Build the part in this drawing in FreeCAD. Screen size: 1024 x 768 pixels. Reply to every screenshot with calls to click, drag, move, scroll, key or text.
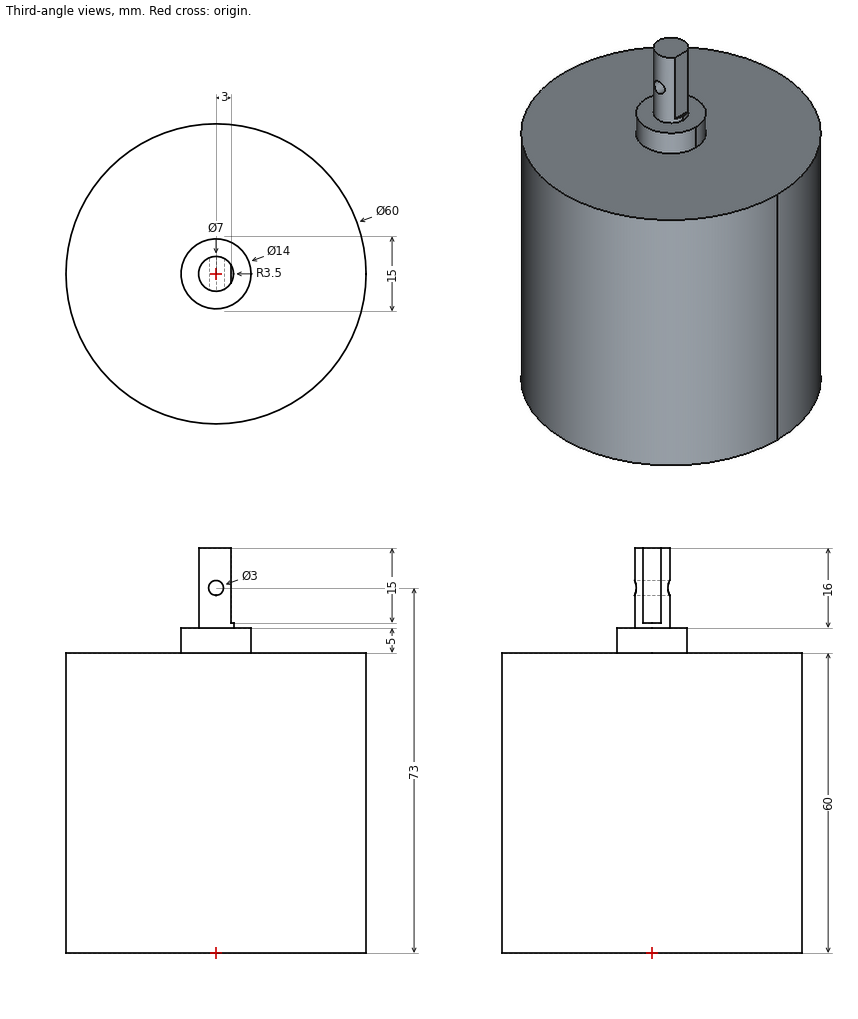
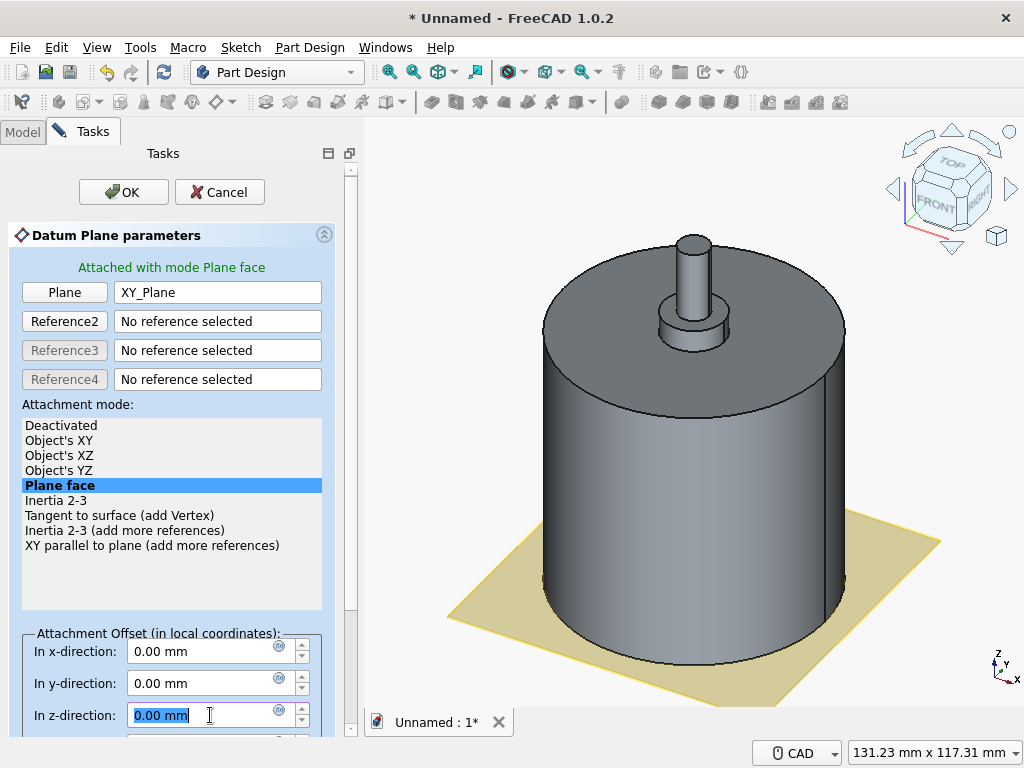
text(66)
key(Tab)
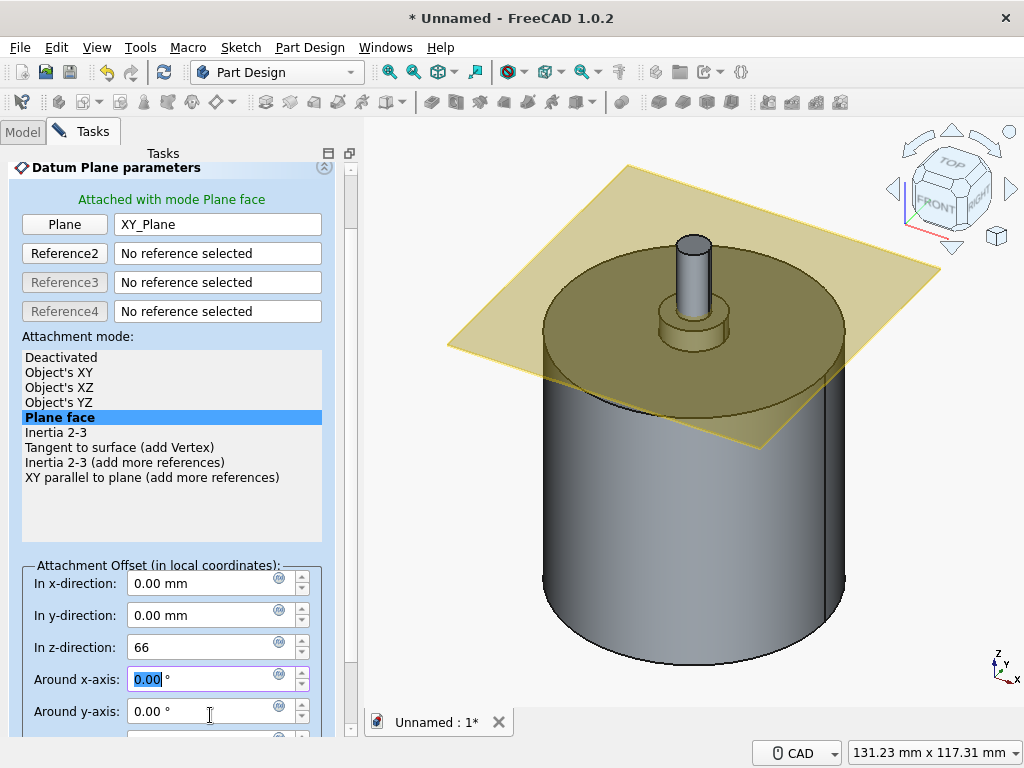
scroll(351, 450, up, 2)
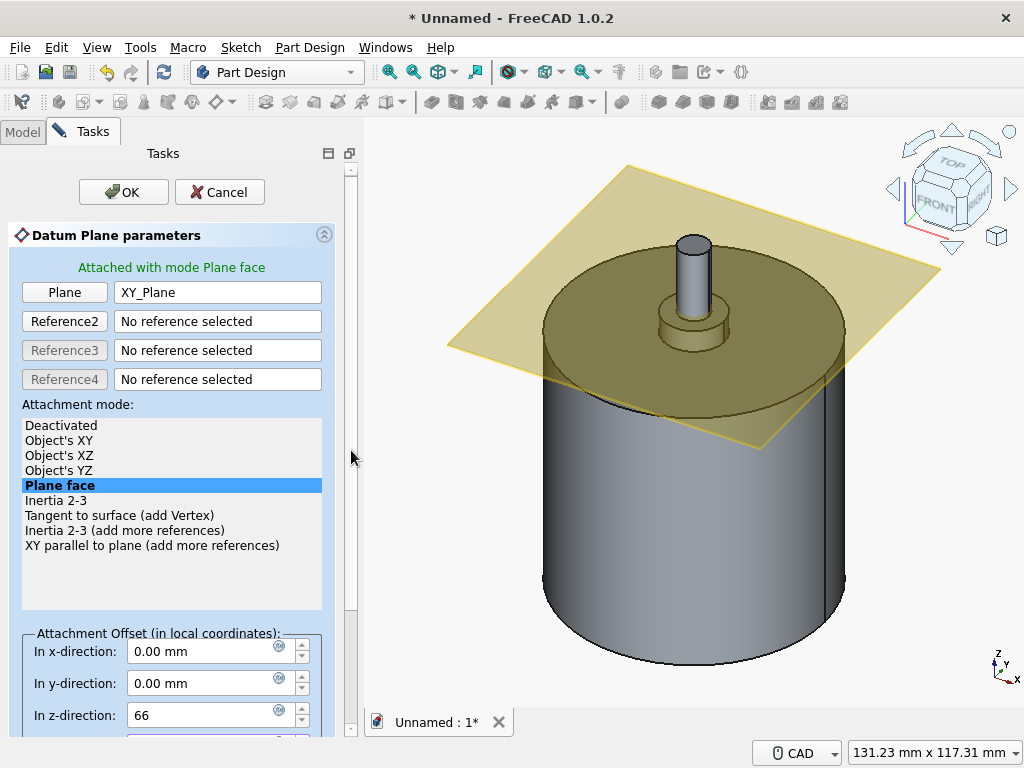
click(124, 192)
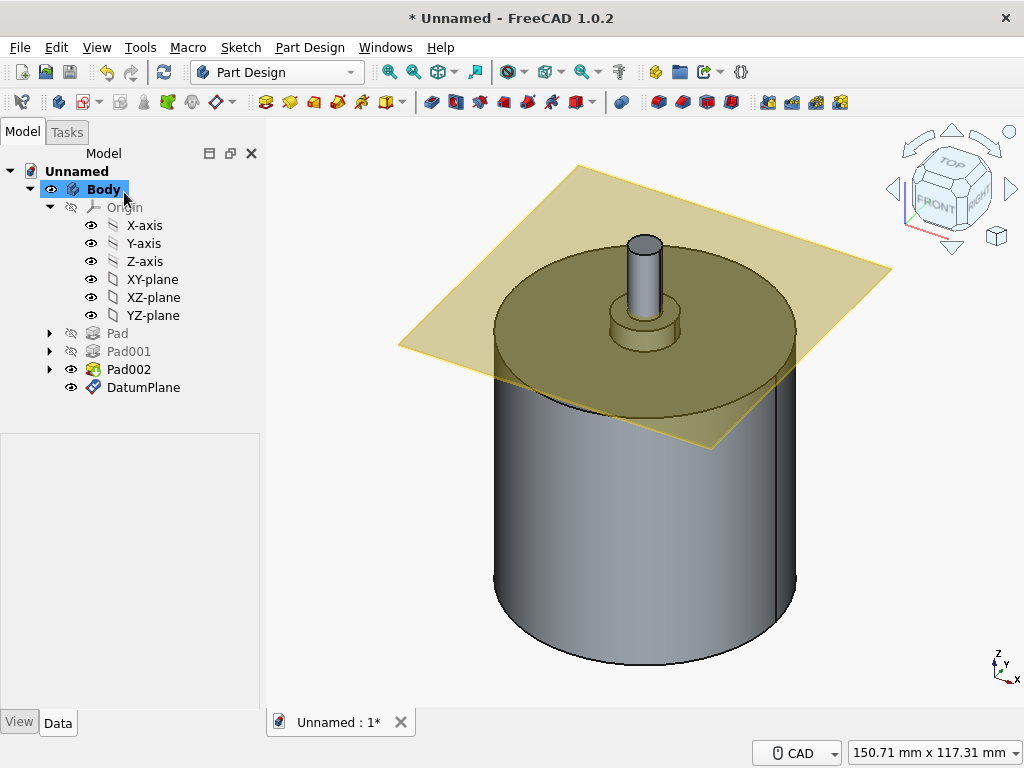
click(116, 387)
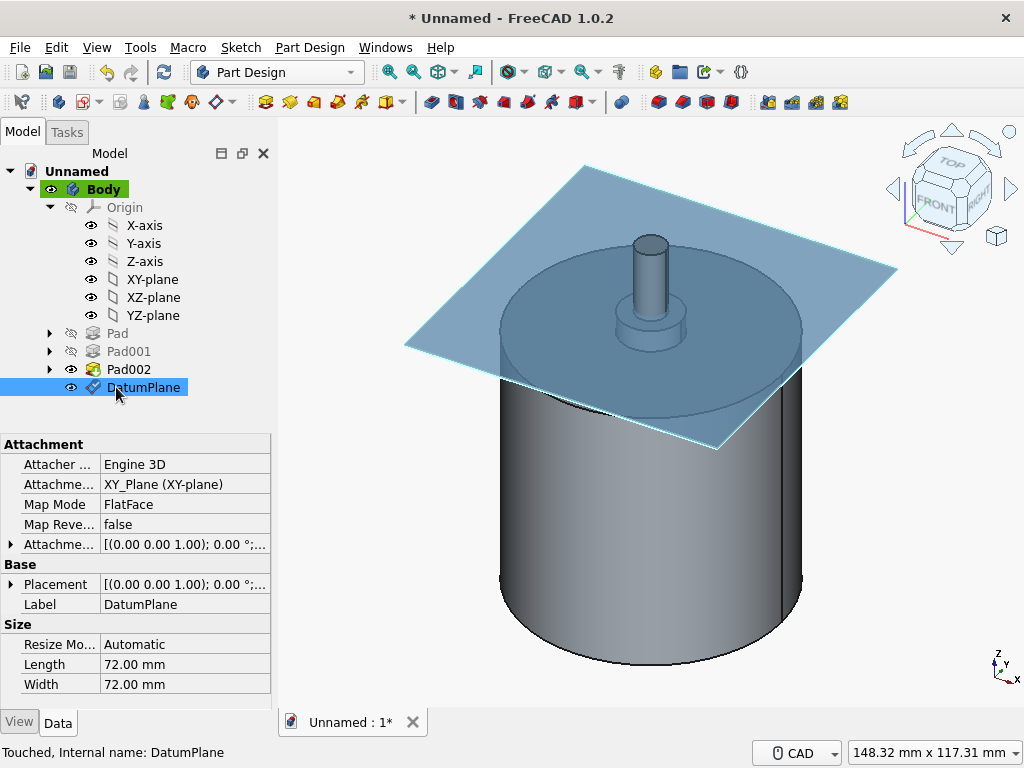
click(84, 102)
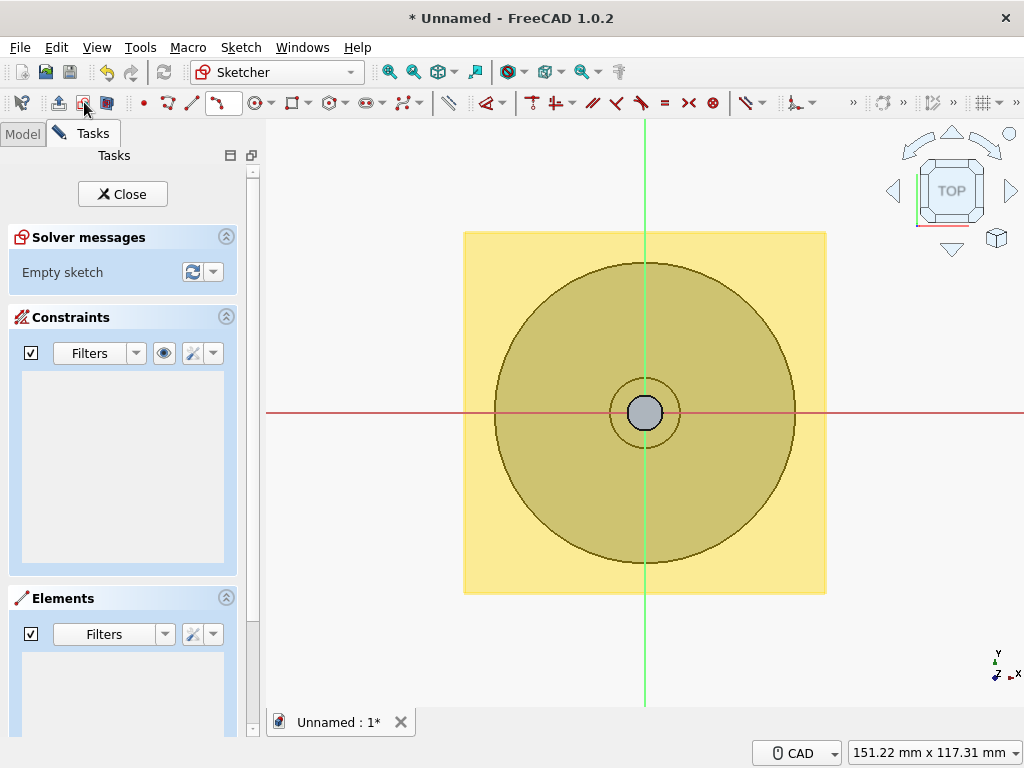
click(108, 104)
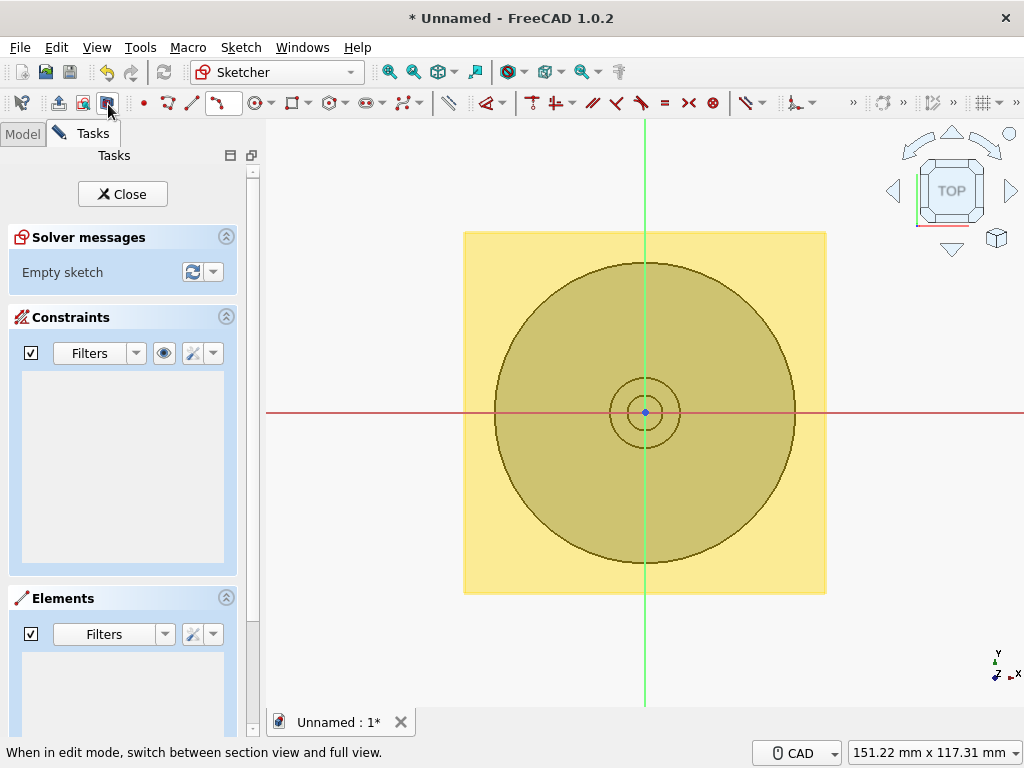
scroll(658, 413, up, 15)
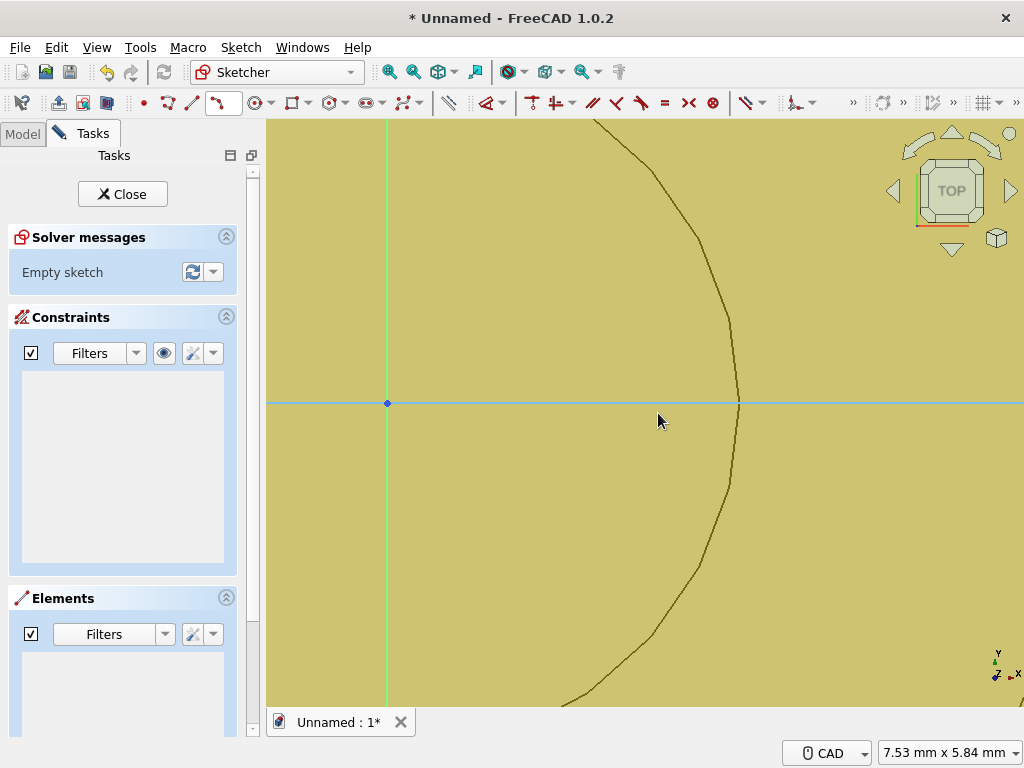
click(192, 104)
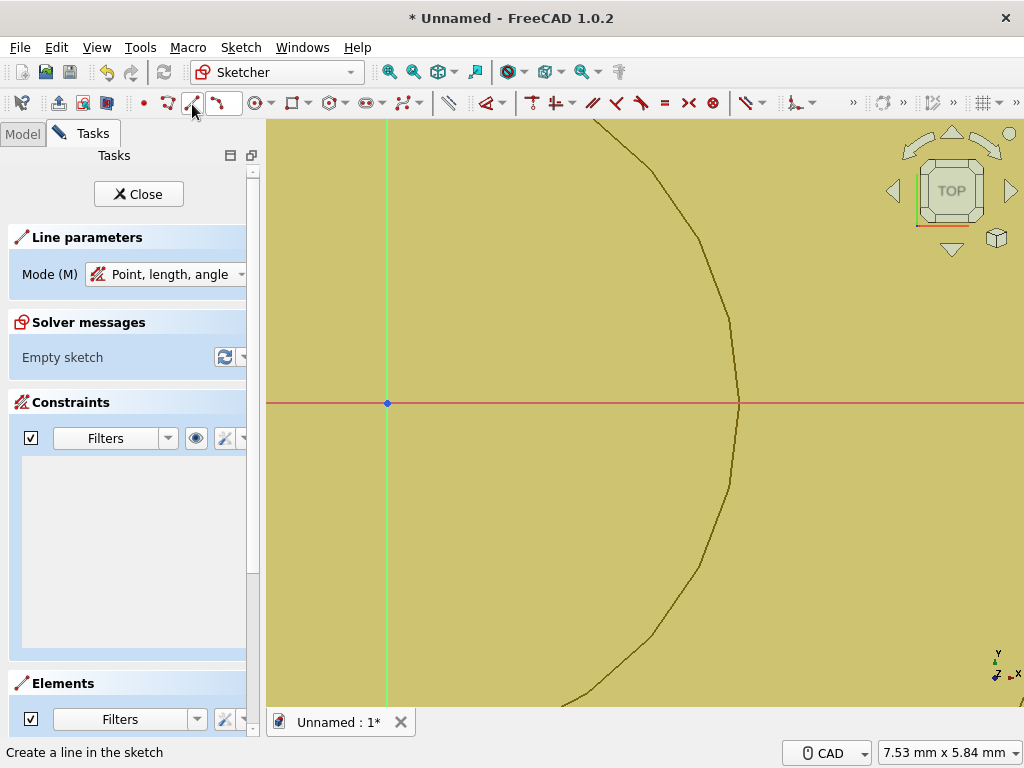
click(689, 222)
click(689, 585)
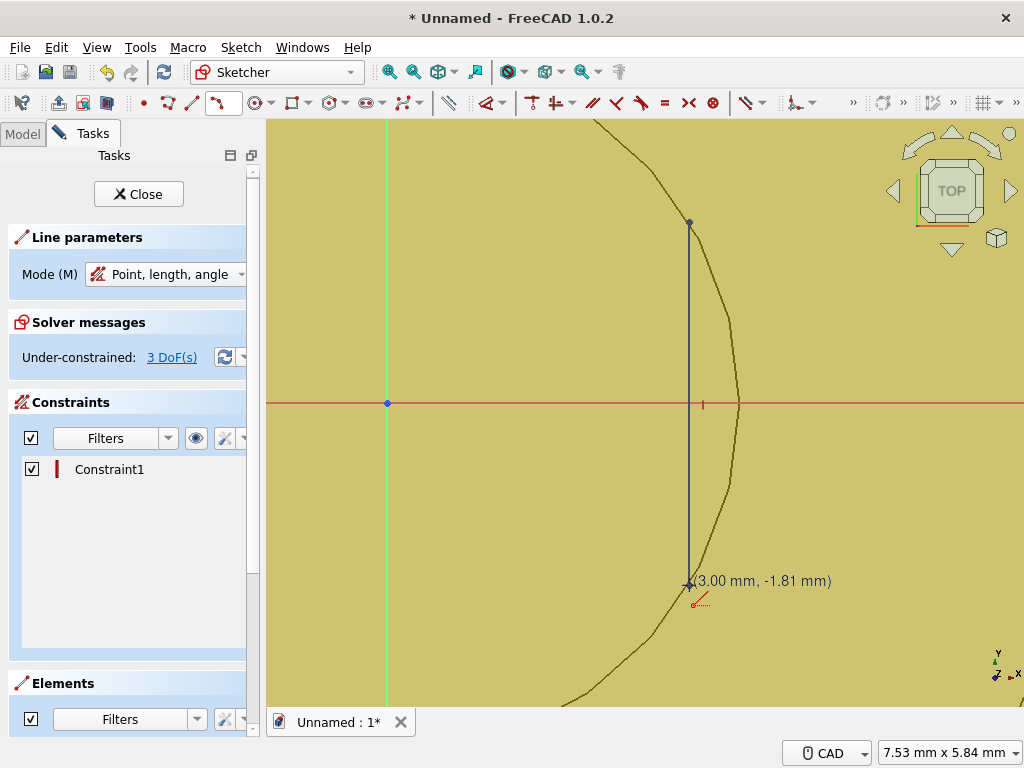
click(218, 104)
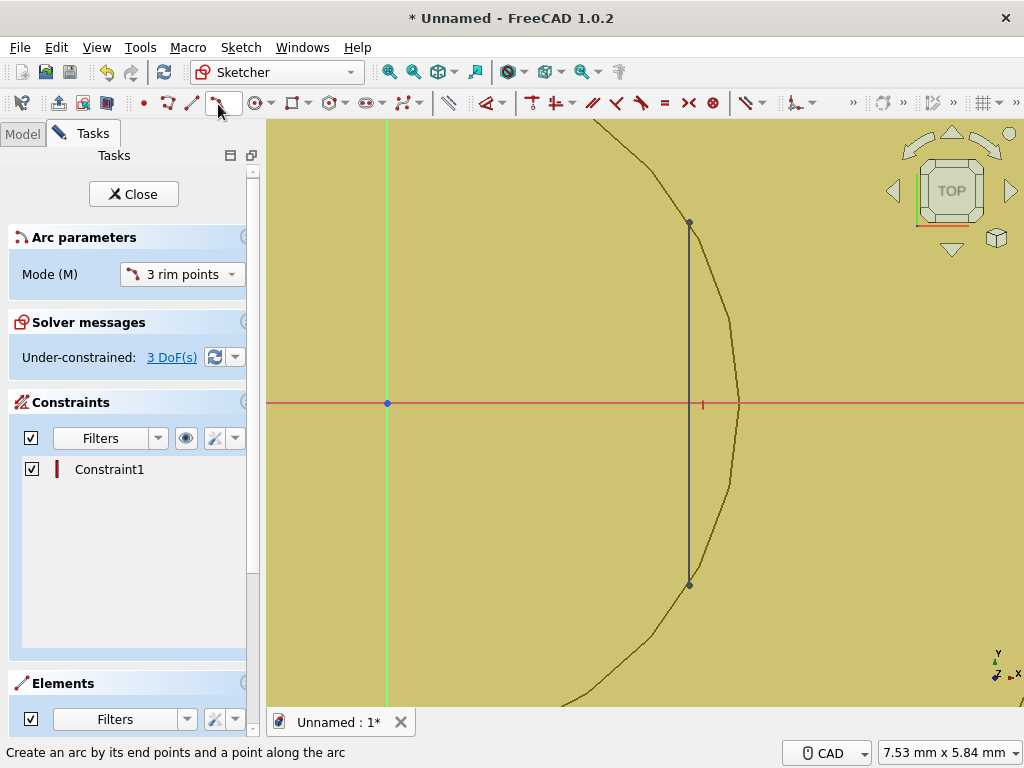
click(689, 586)
click(689, 223)
click(737, 442)
key(Escape)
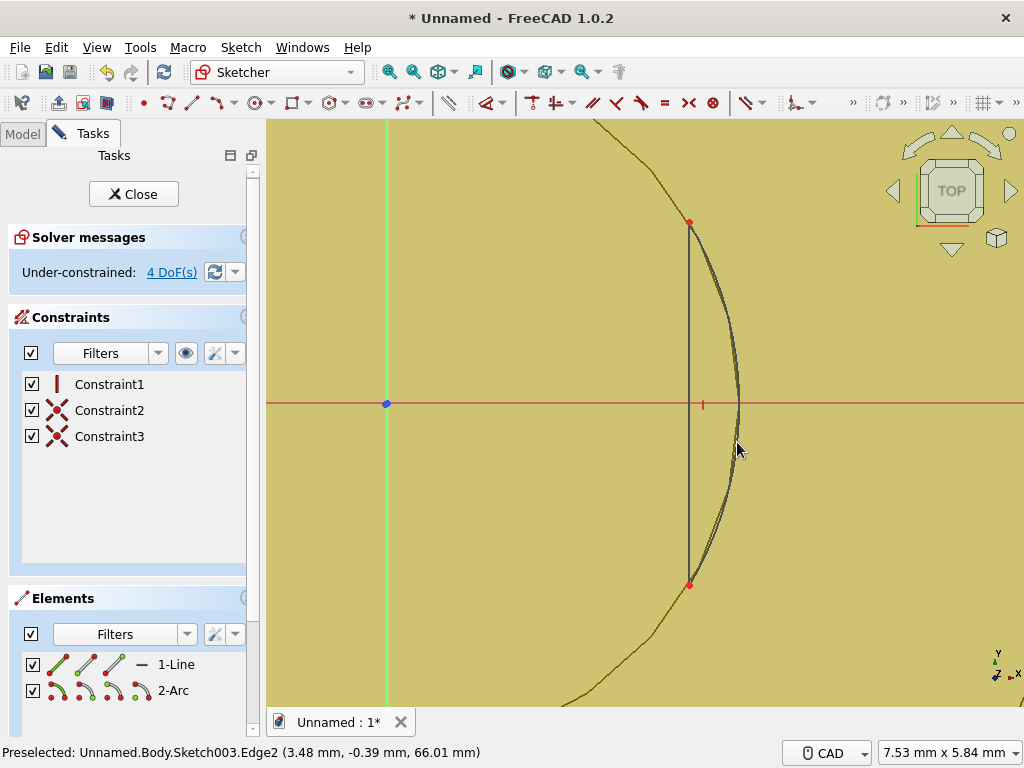
drag(375, 393, 397, 414)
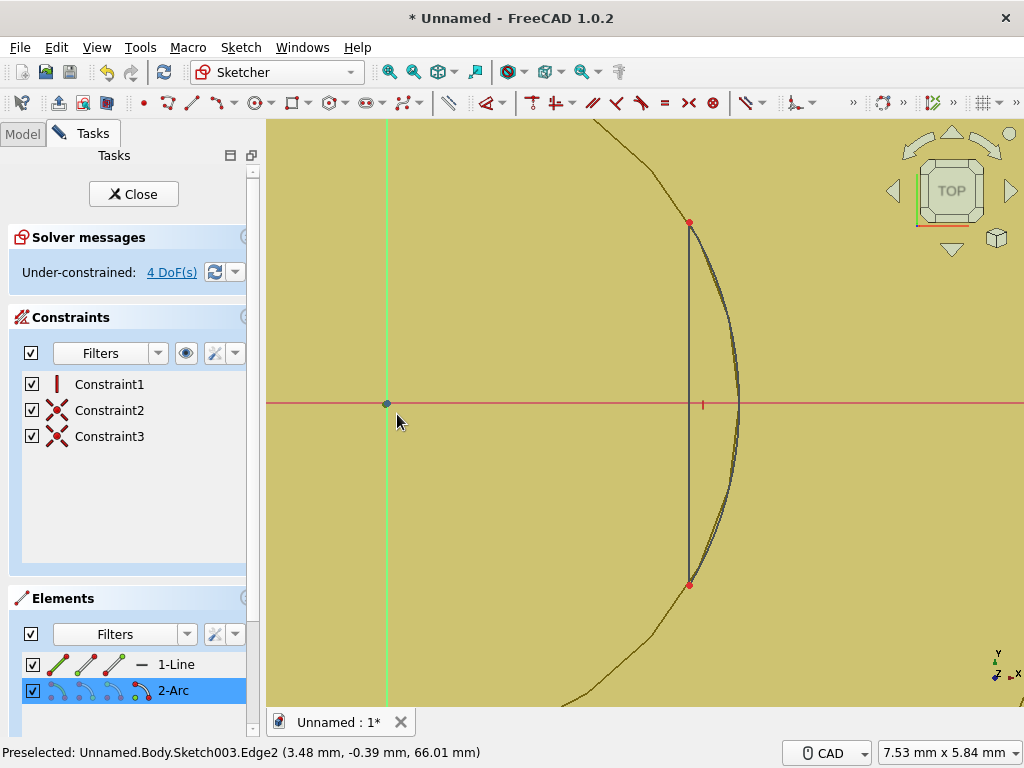
click(532, 104)